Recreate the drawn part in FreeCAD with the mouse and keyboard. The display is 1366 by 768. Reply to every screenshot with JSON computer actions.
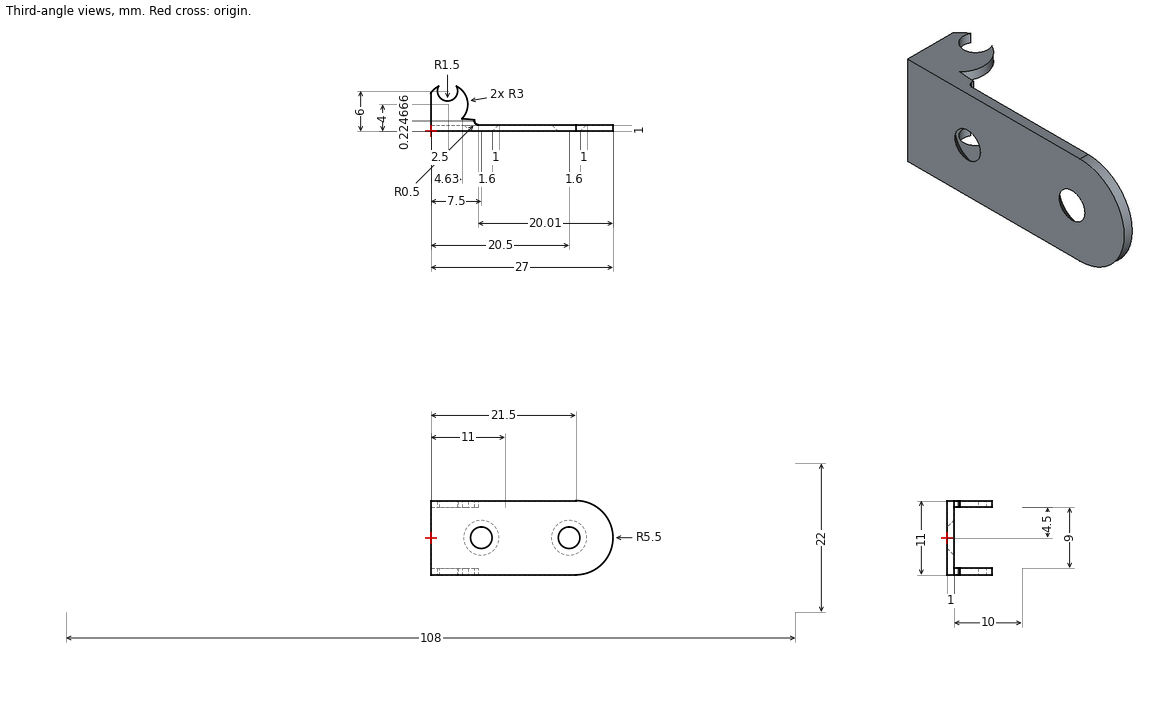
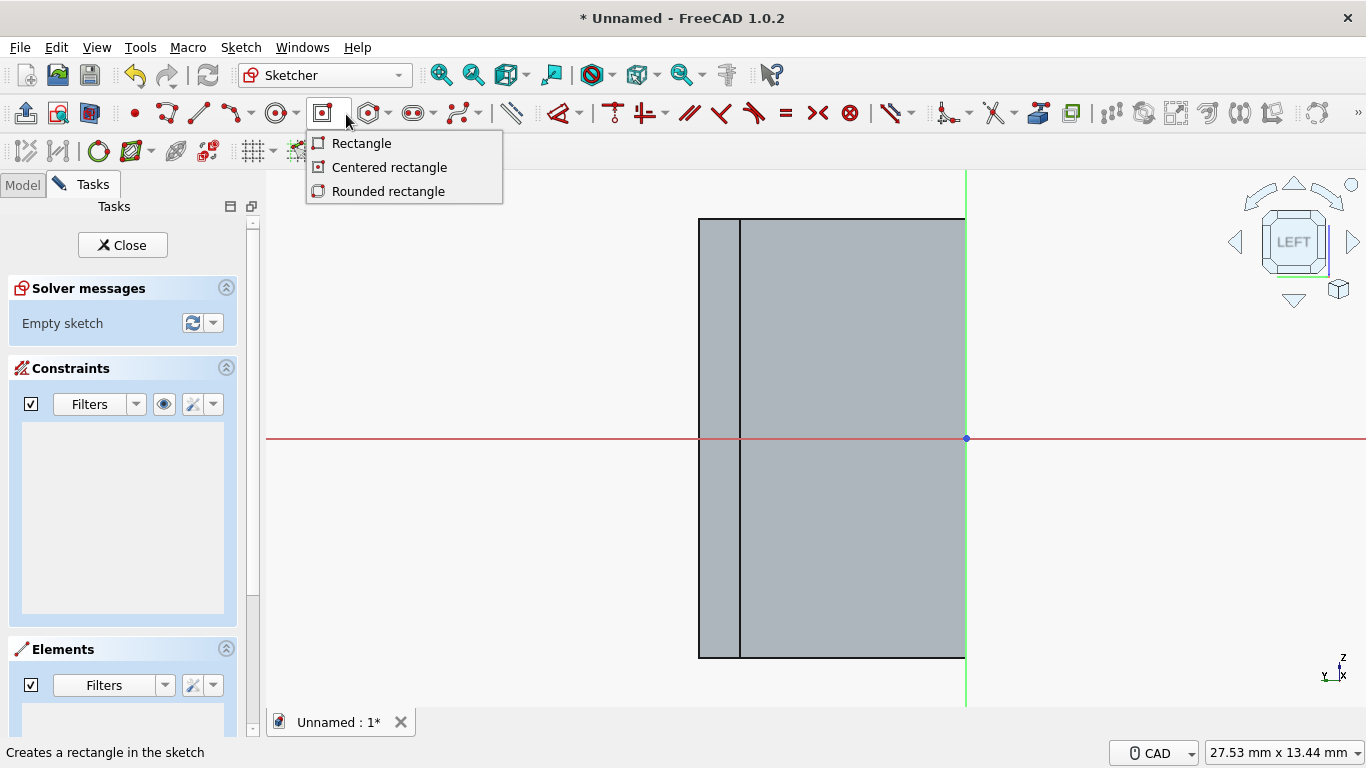
{"action": "left_click", "coordinate": [404, 143]}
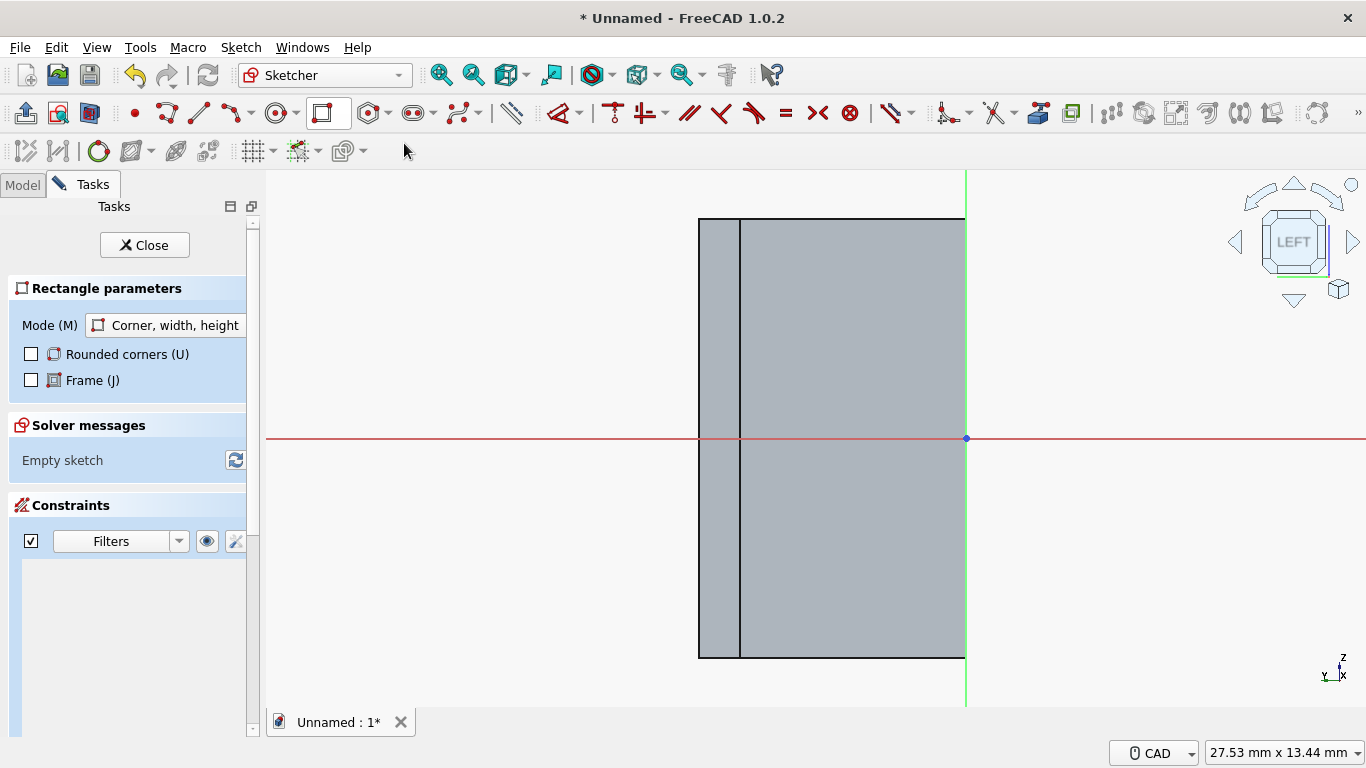
{"action": "left_click", "coordinate": [527, 259]}
{"action": "left_click", "coordinate": [926, 618]}
{"action": "key", "text": "Escape"}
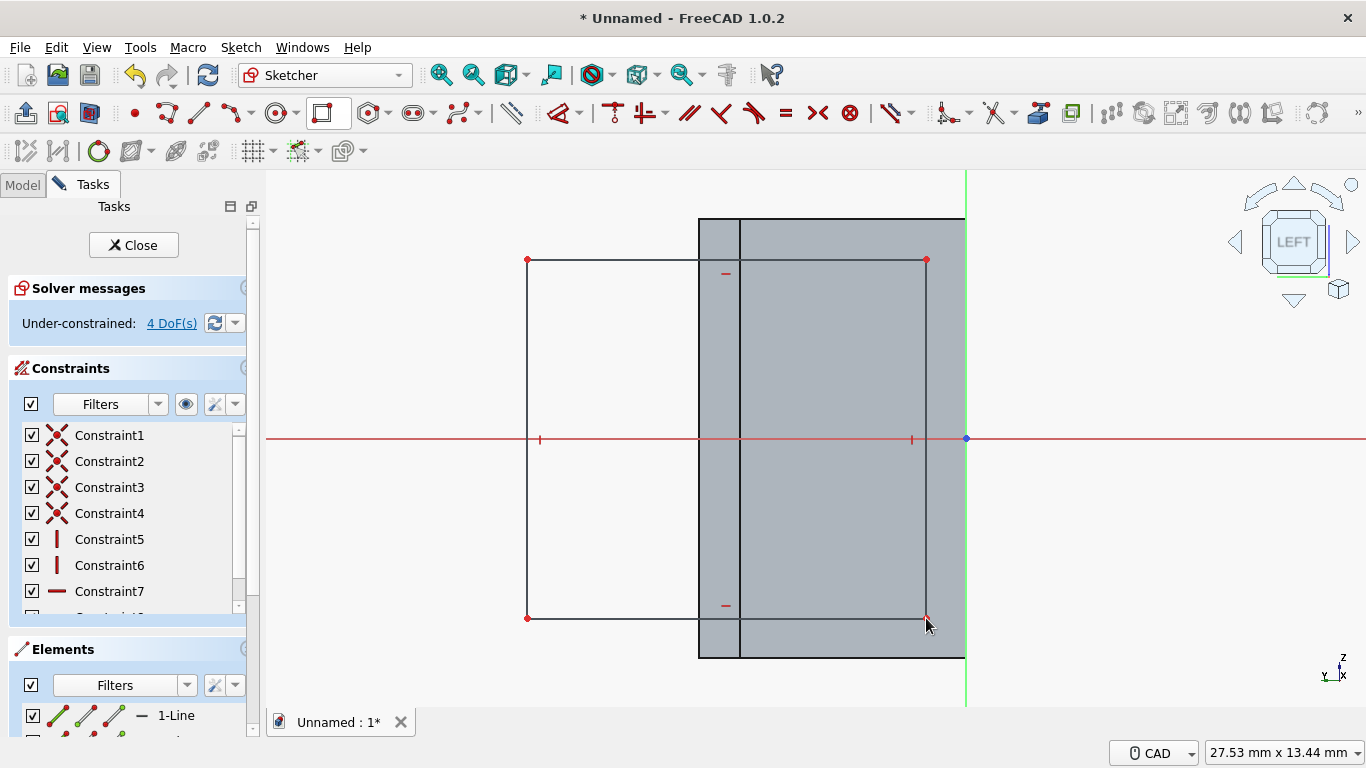
{"action": "left_click", "coordinate": [558, 114]}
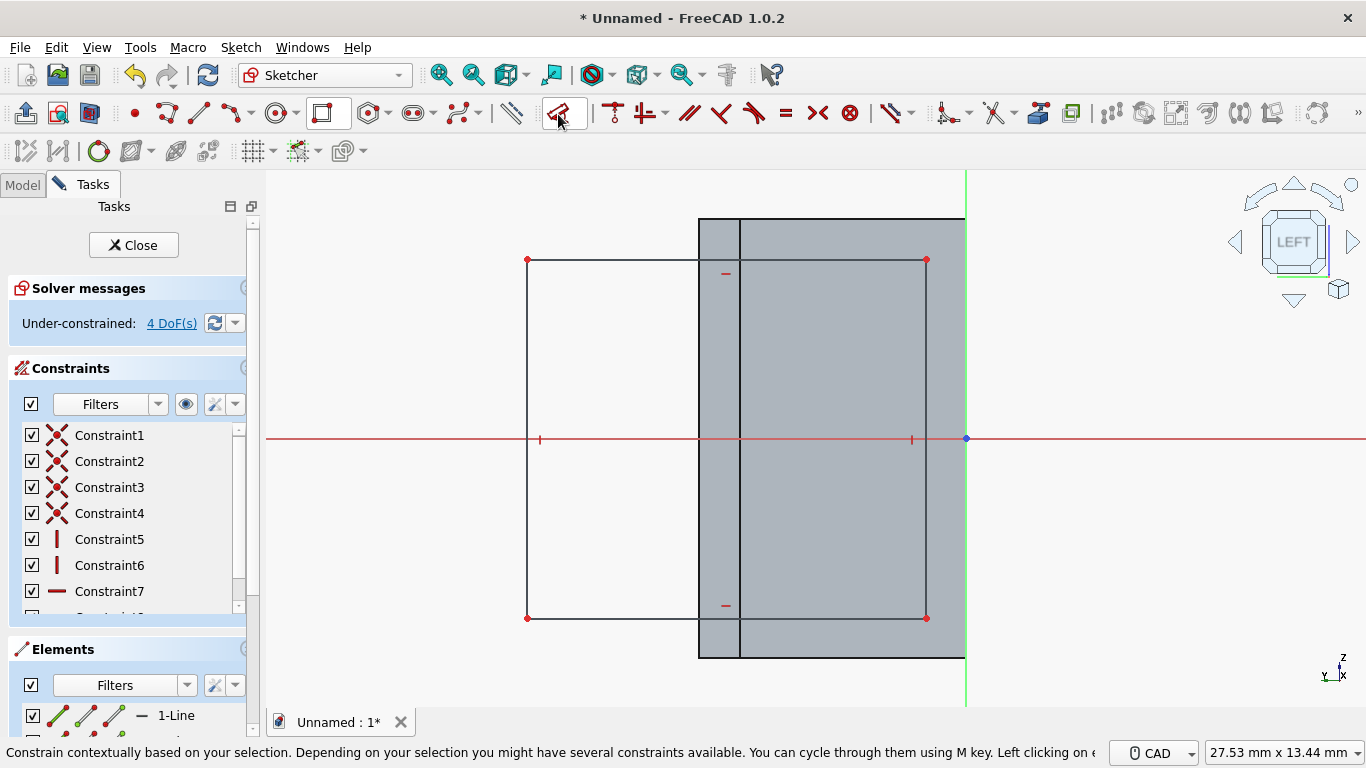
{"action": "left_click", "coordinate": [527, 368]}
{"action": "left_click", "coordinate": [493, 357]}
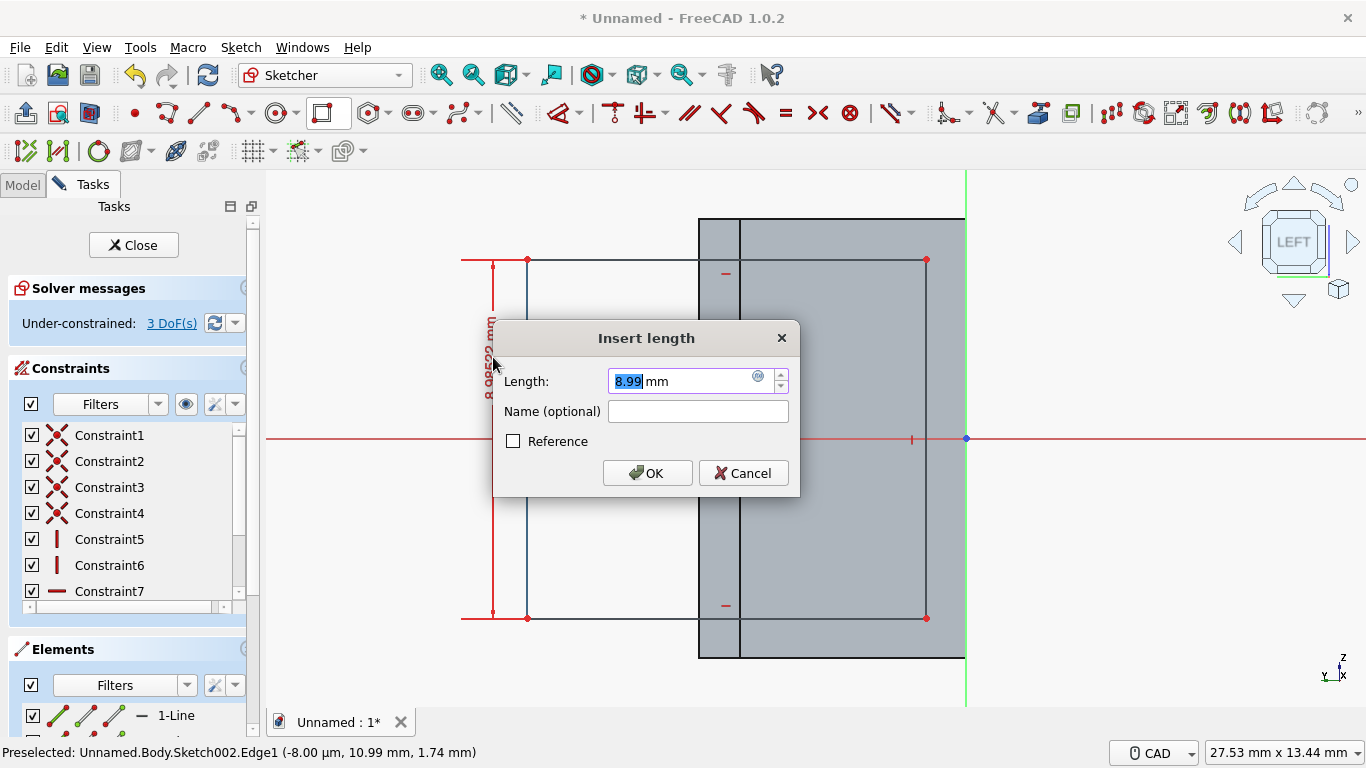
{"action": "type", "text": "9"}
{"action": "key", "text": "Return"}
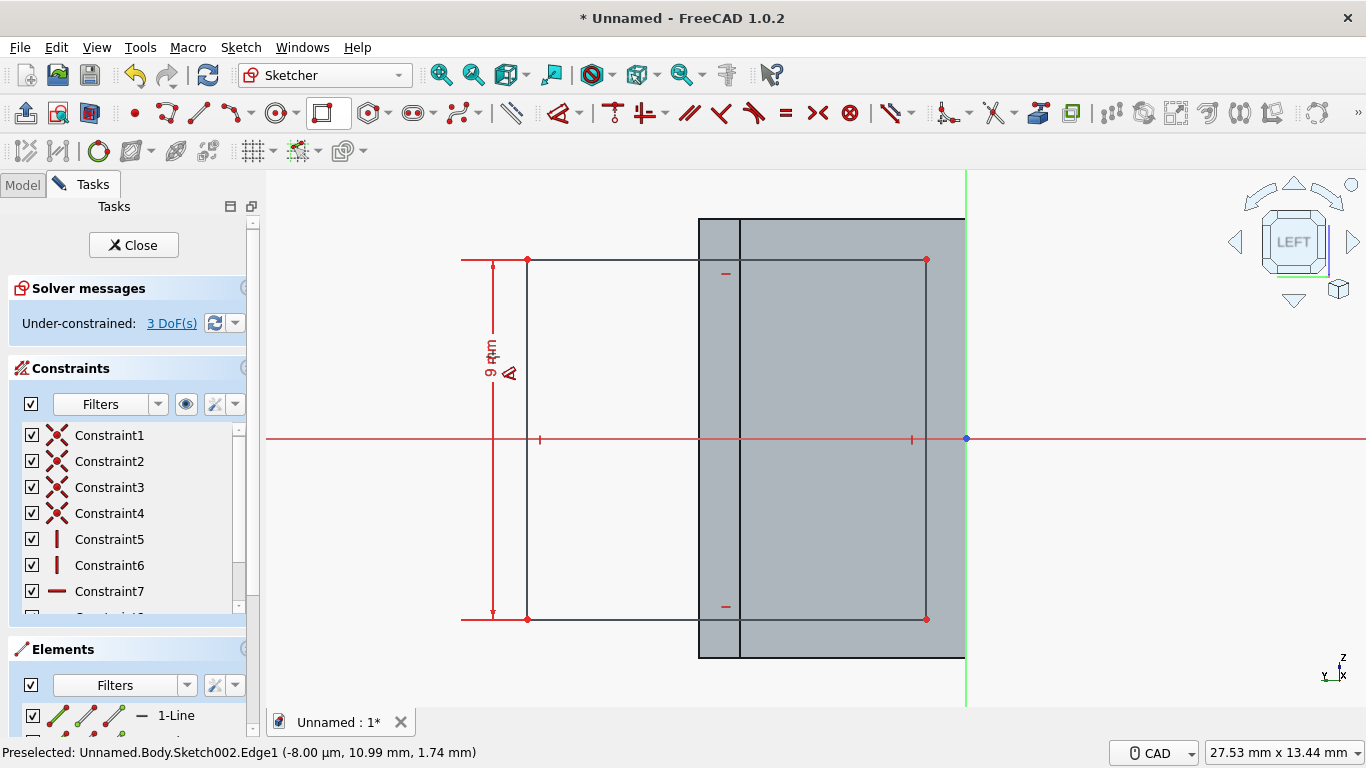
{"action": "left_click", "coordinate": [647, 620]}
{"action": "left_click", "coordinate": [727, 654]}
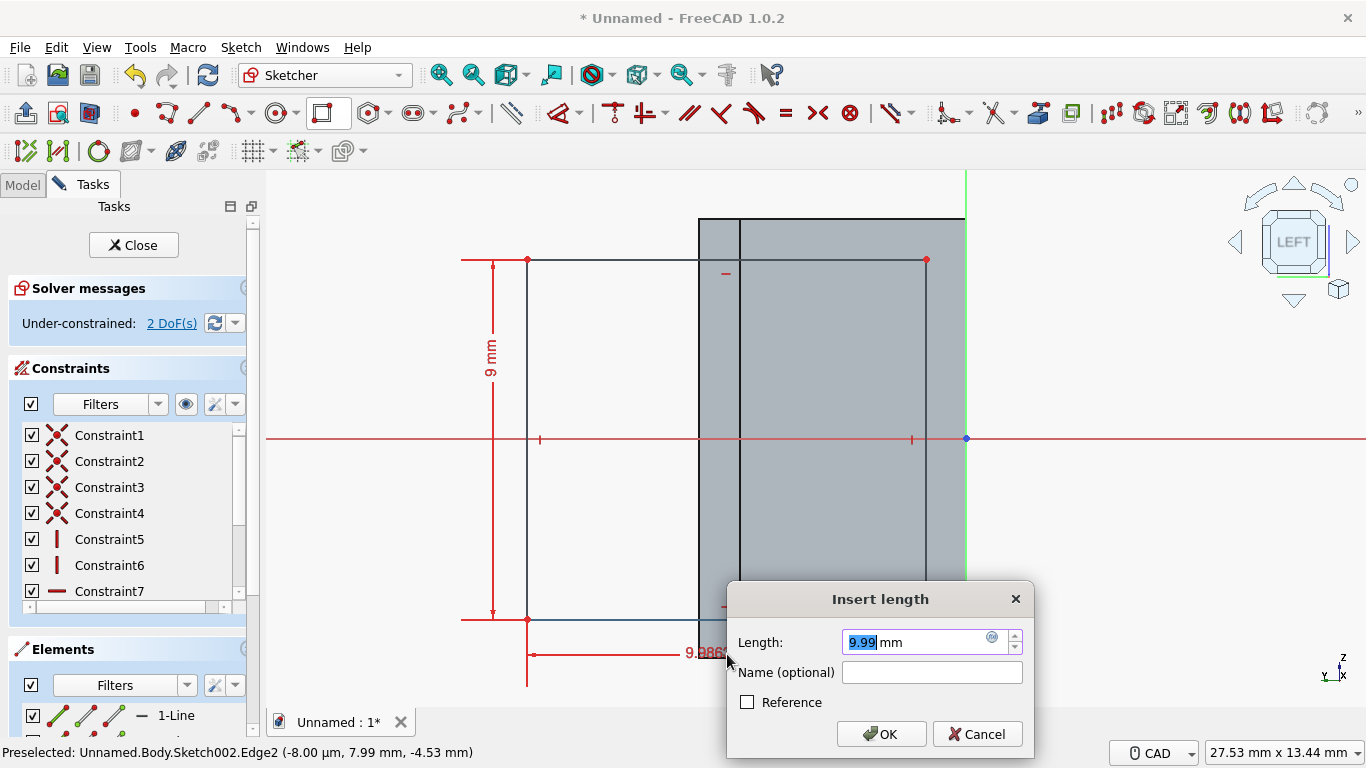
{"action": "type", "text": "10"}
{"action": "key", "text": "Return"}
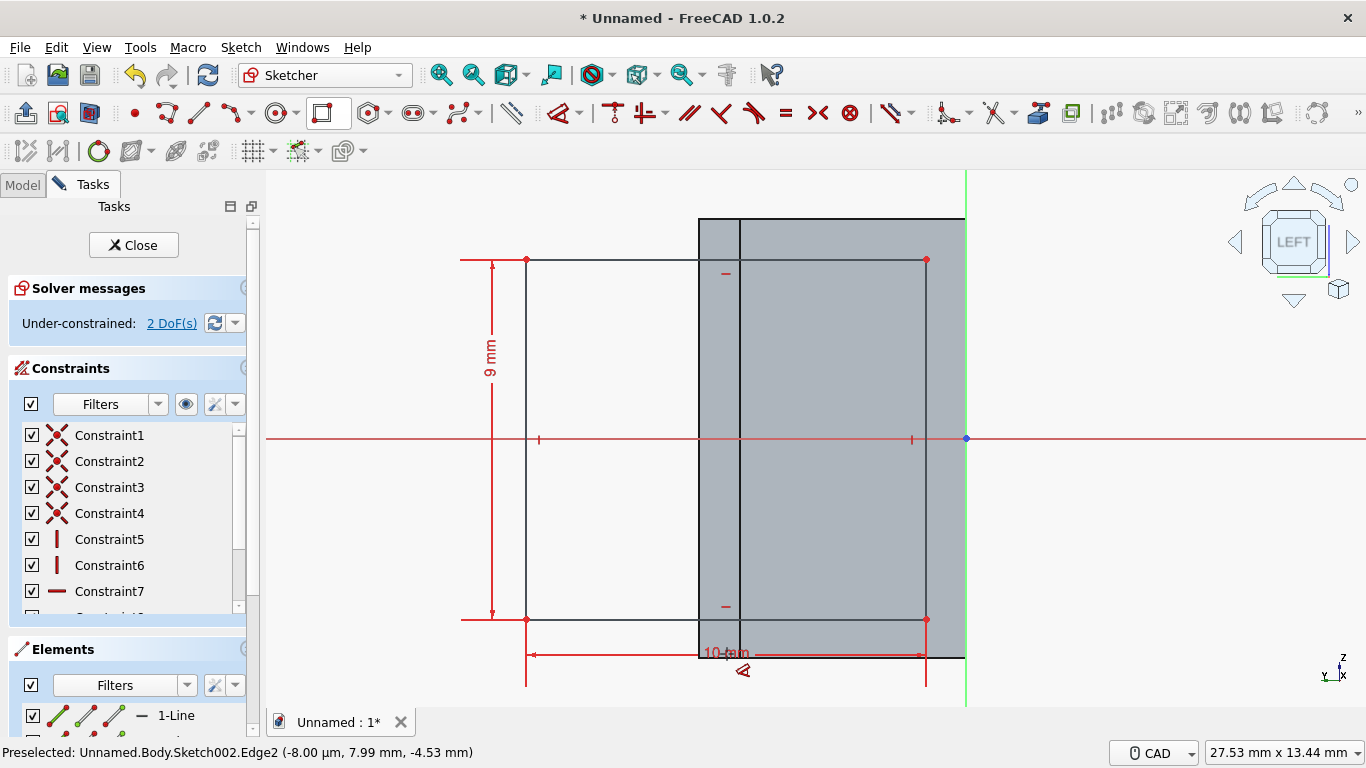
{"action": "left_click", "coordinate": [926, 620]}
{"action": "left_click", "coordinate": [946, 654]}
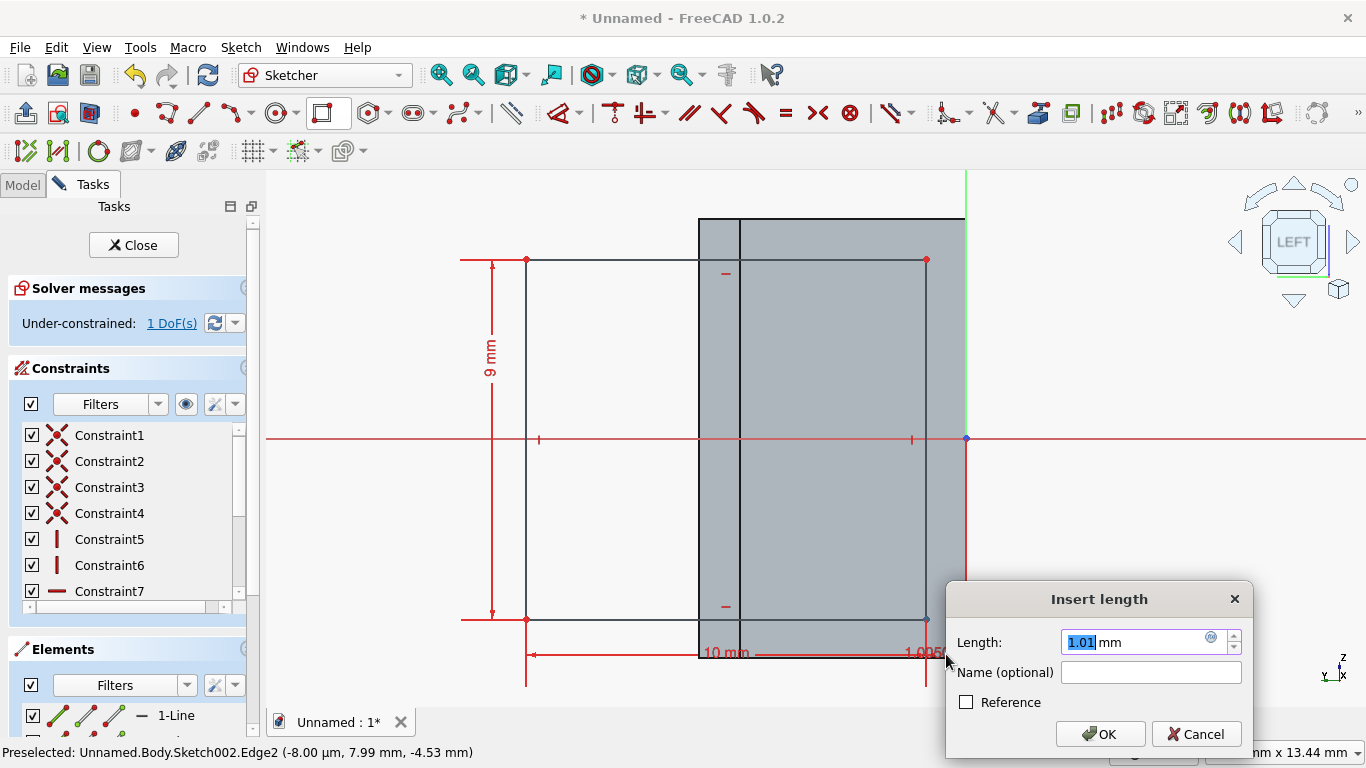
{"action": "type", "text": "1"}
{"action": "key", "text": "Return"}